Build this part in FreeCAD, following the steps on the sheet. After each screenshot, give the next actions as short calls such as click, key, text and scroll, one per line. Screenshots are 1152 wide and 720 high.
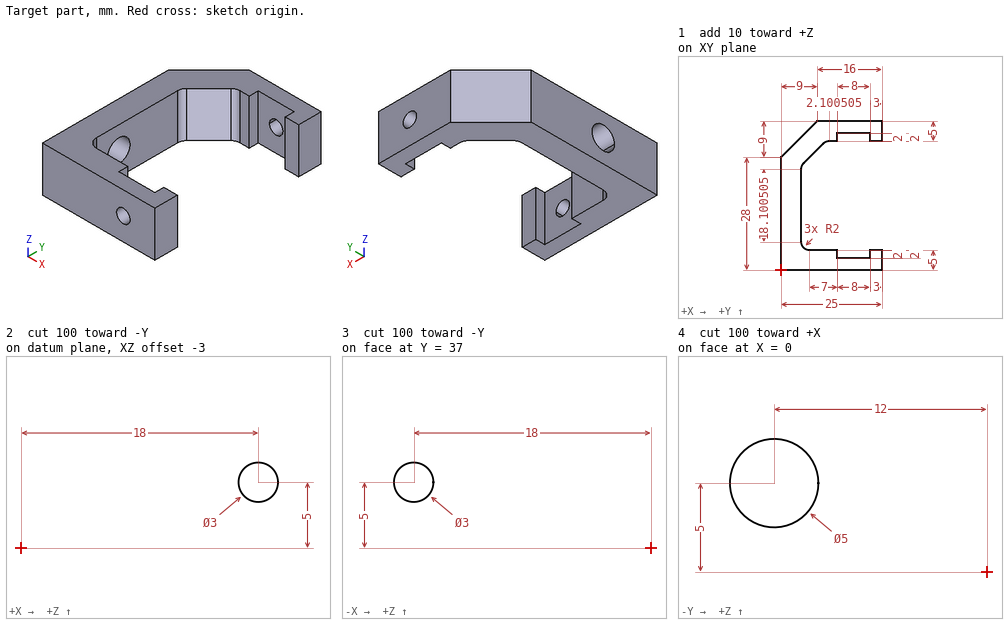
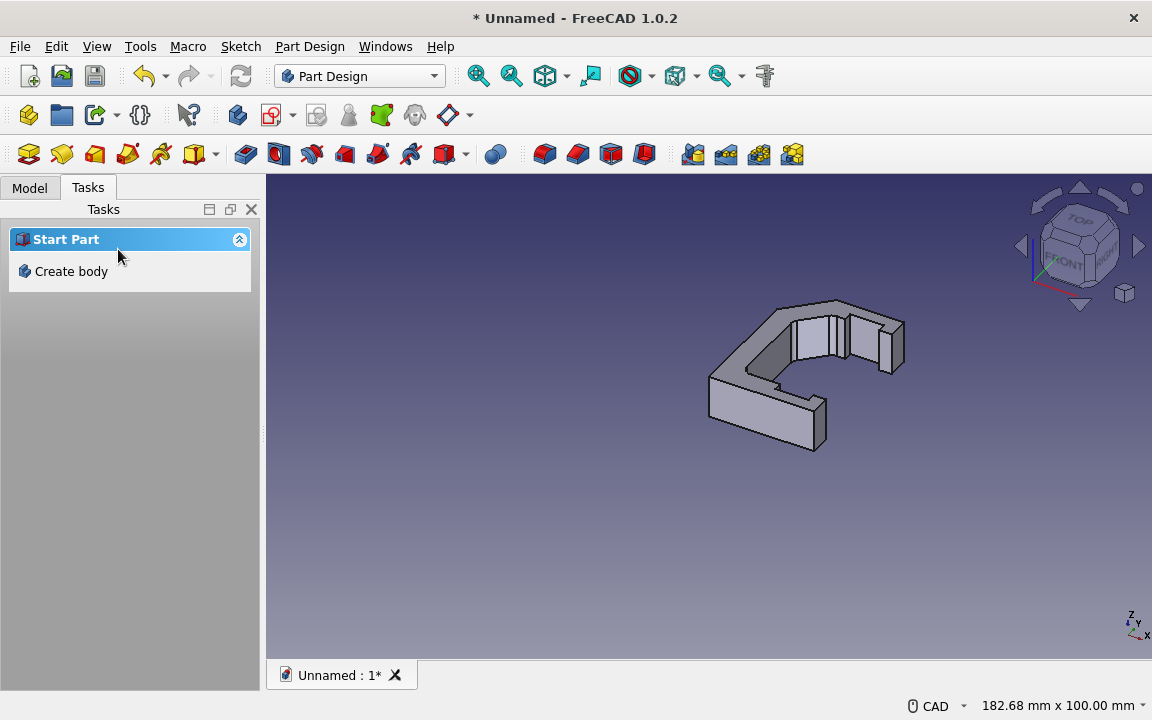
click(479, 76)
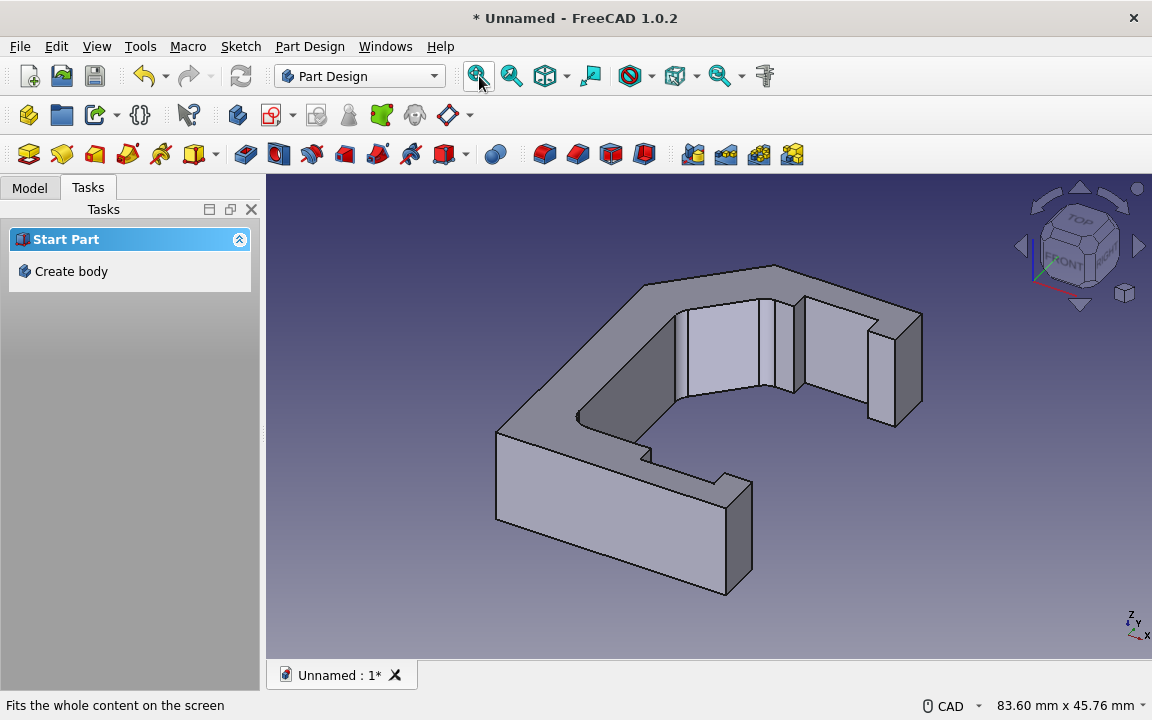
click(30, 188)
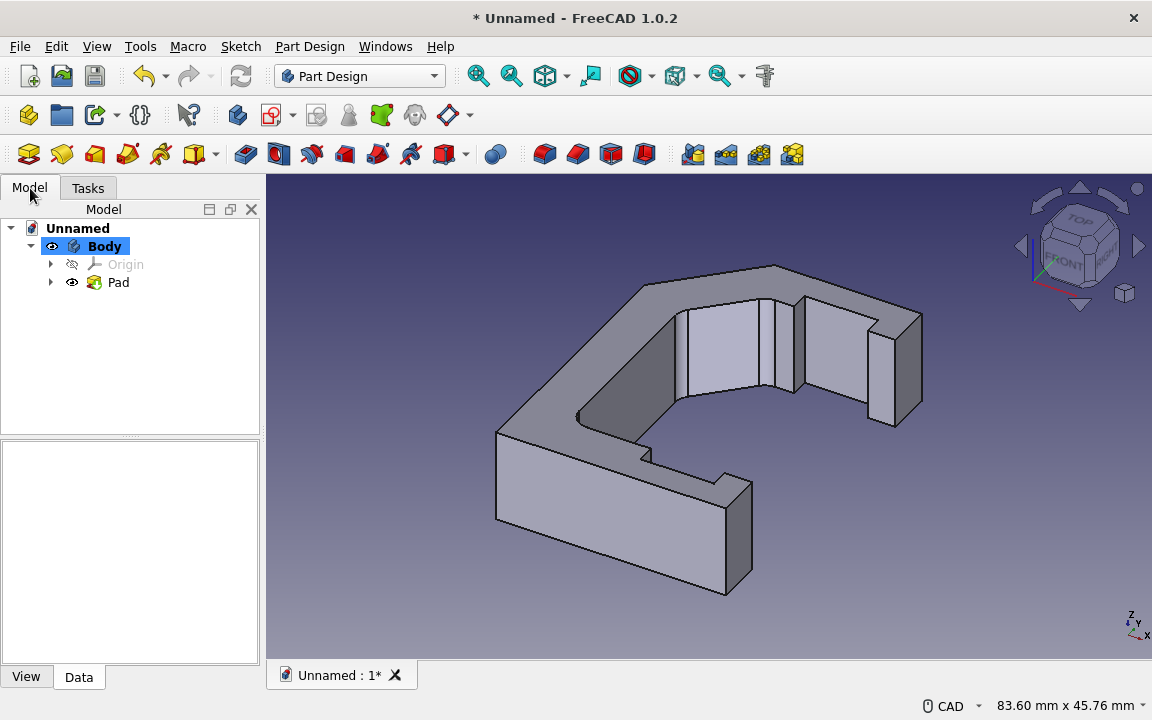
click(51, 264)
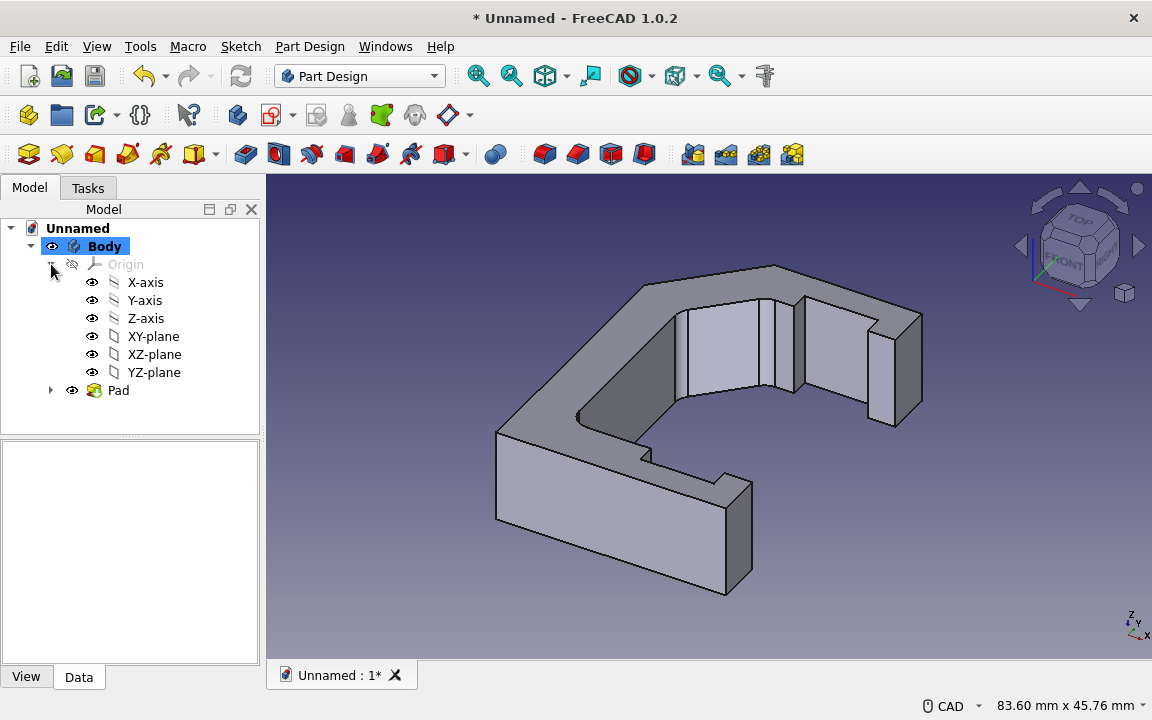
click(137, 354)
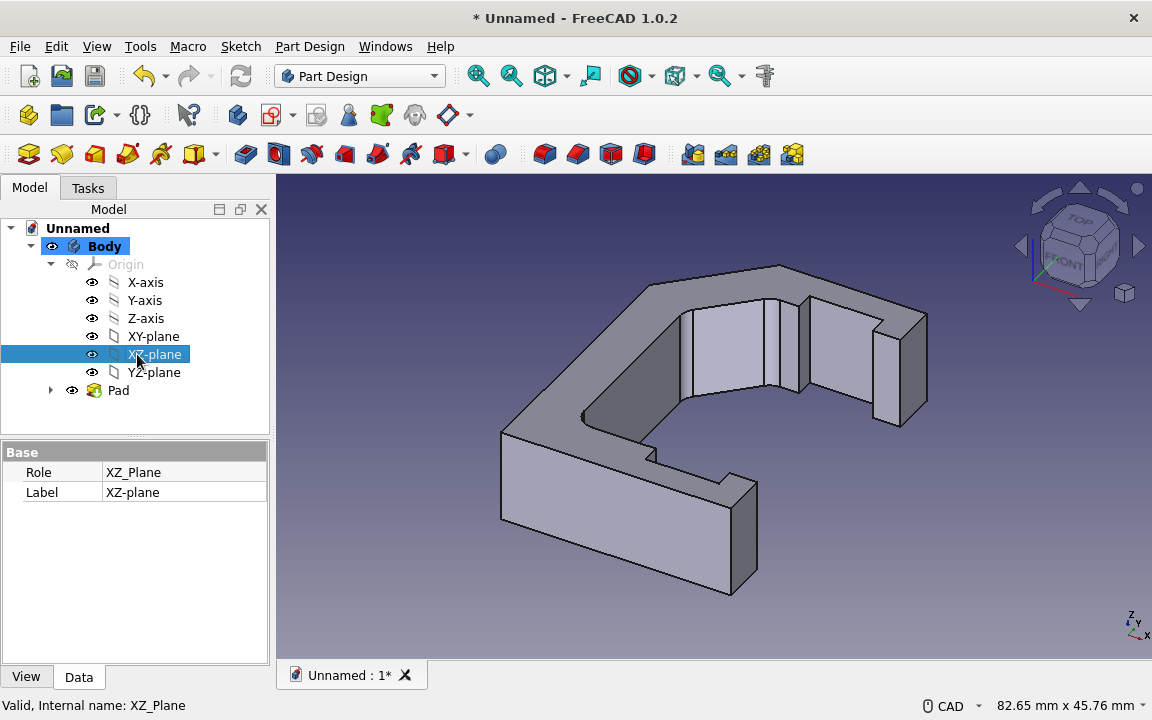
click(448, 116)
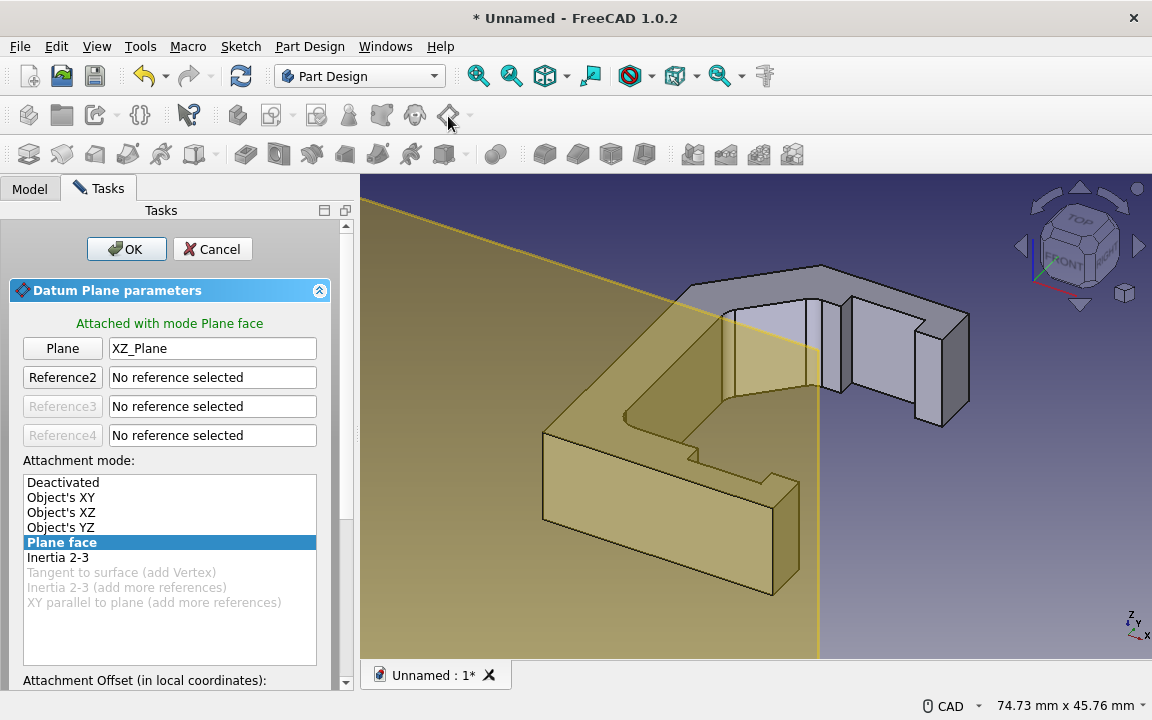
scroll(346, 455, down, 3)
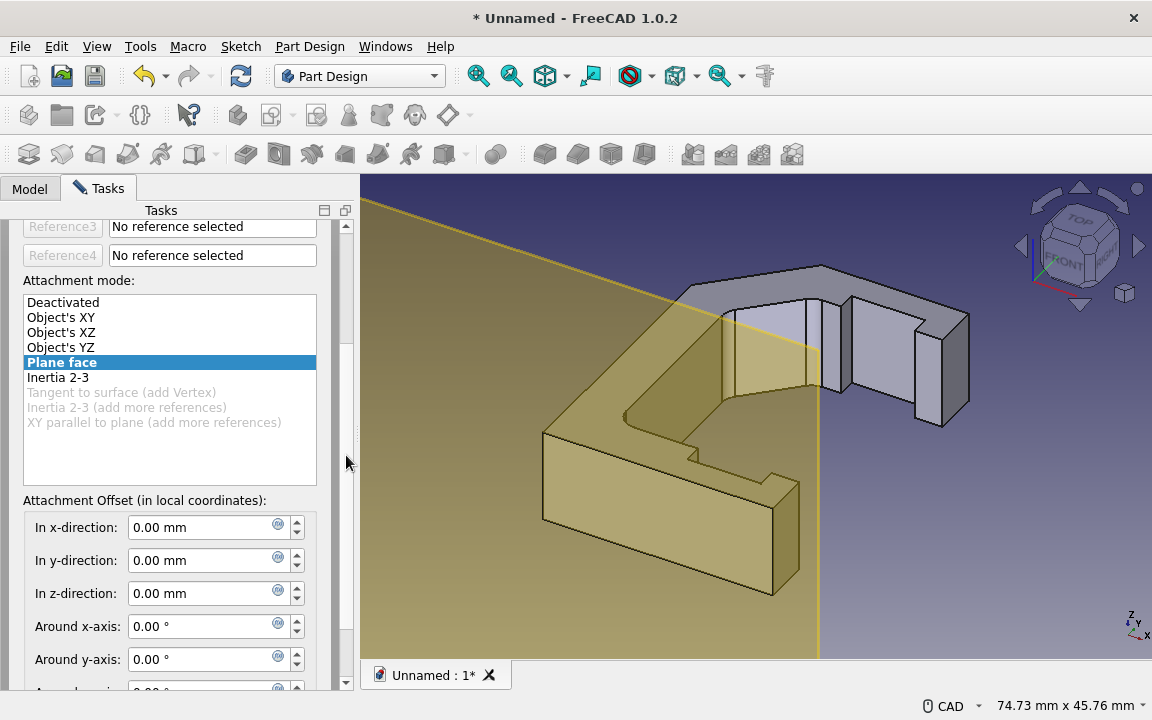
triple_click(210, 594)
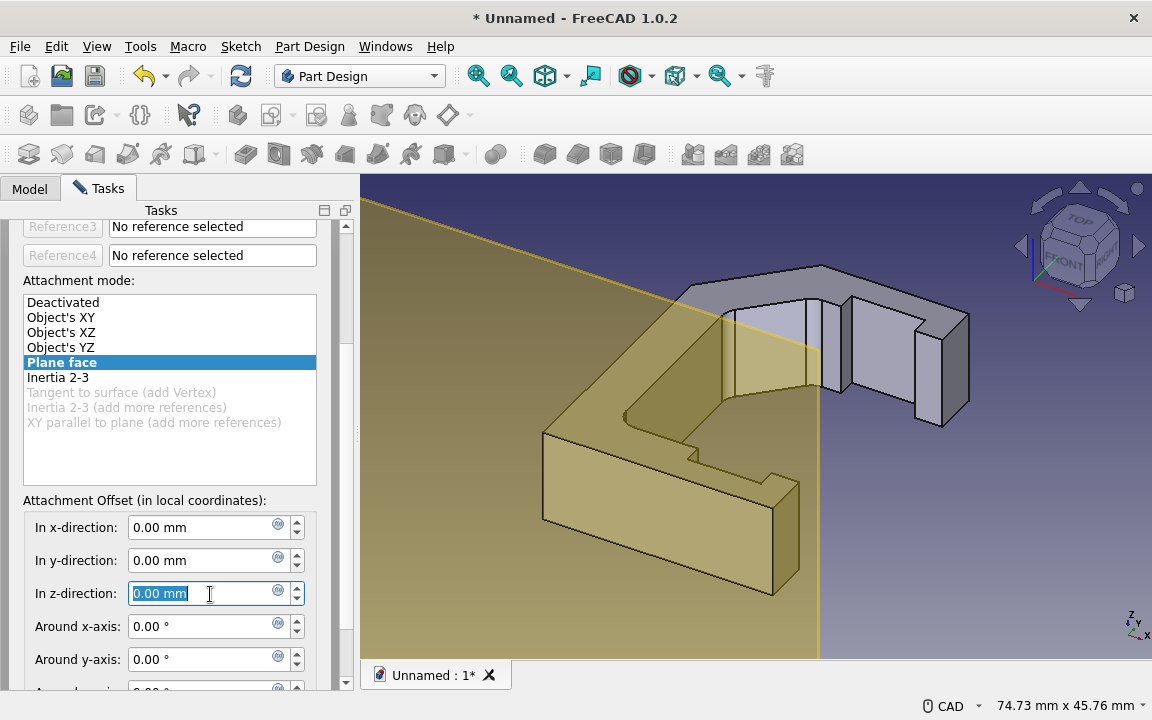
text(-3)
key(Tab)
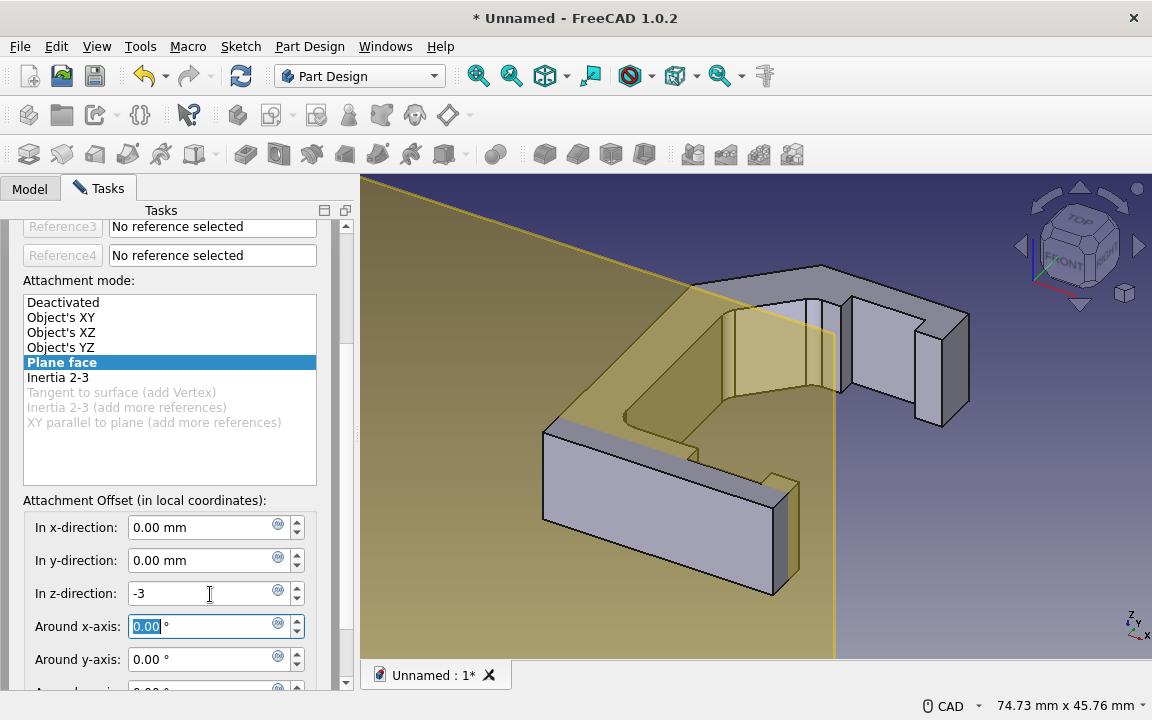
scroll(346, 455, up, 4)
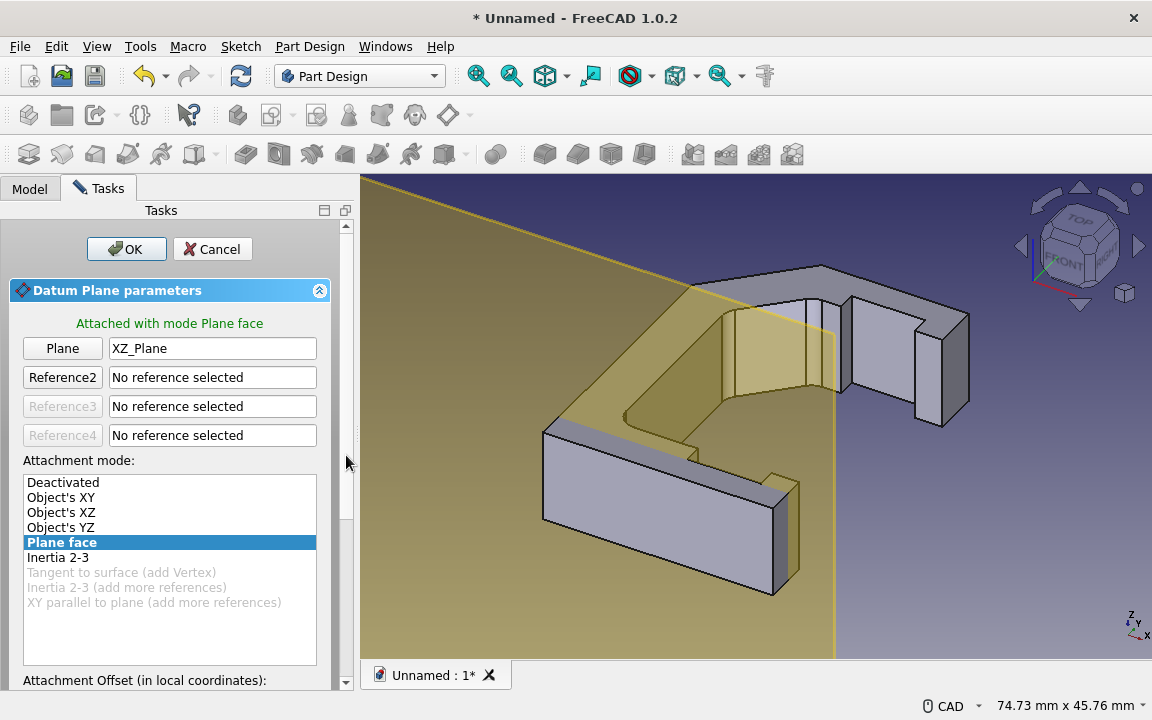
click(127, 249)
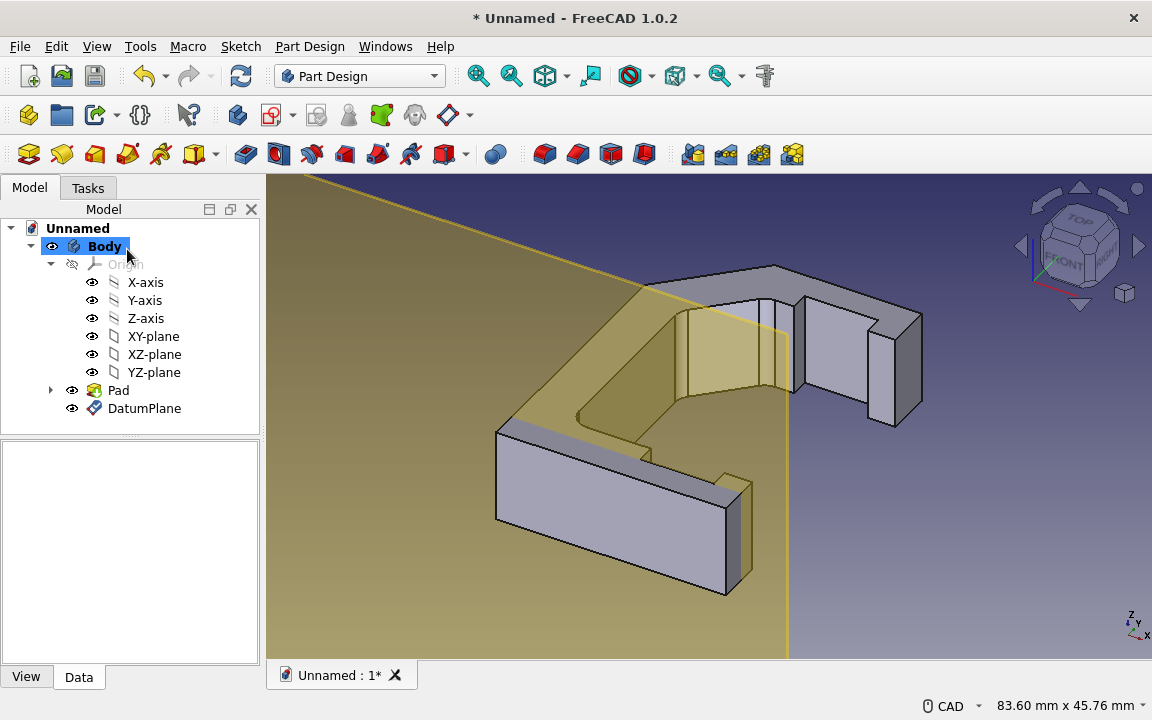
click(117, 408)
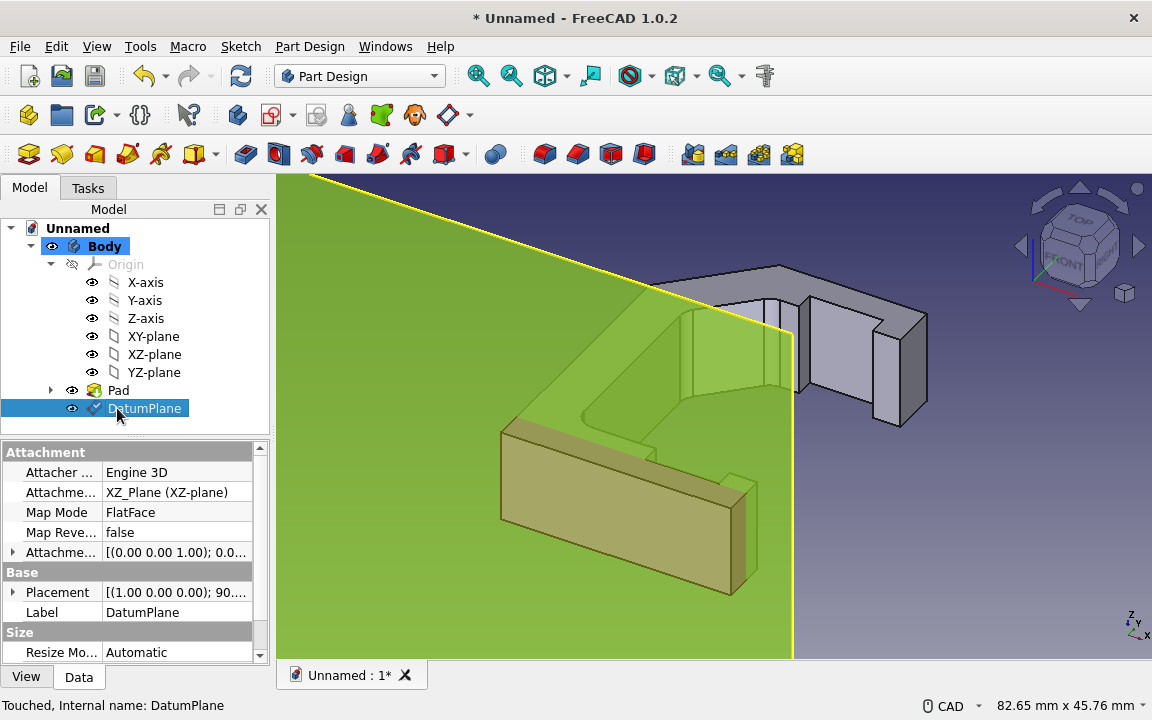
click(270, 116)